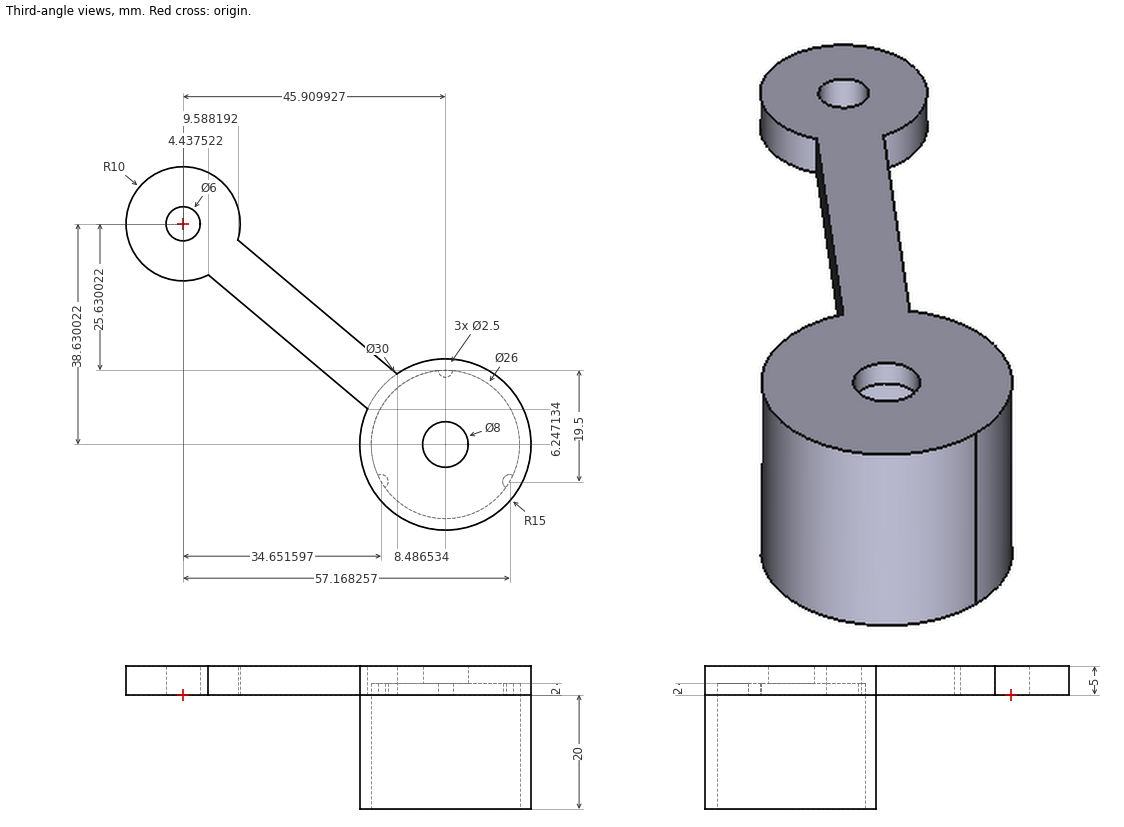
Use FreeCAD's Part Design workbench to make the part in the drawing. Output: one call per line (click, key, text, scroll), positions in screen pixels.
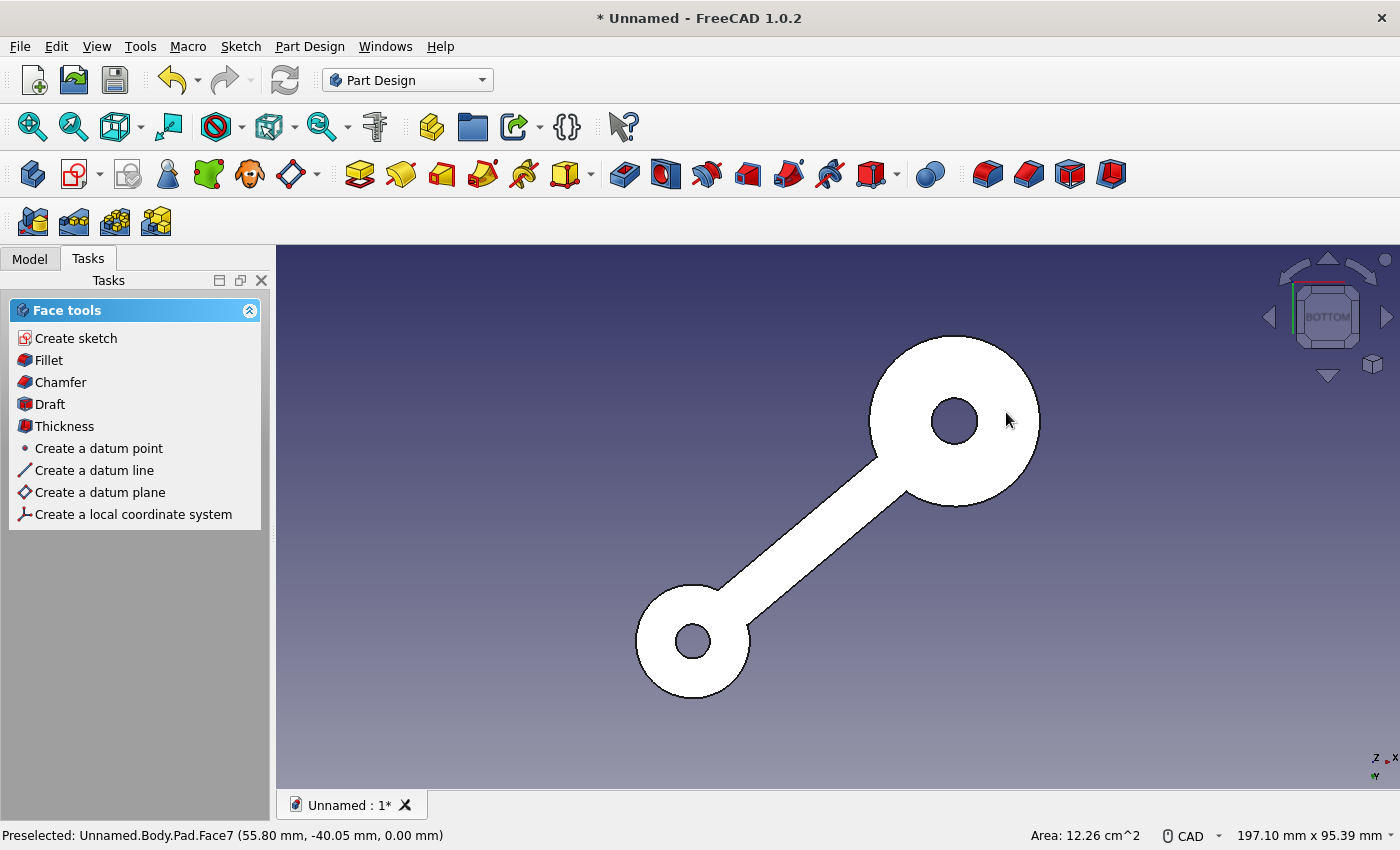
click(74, 174)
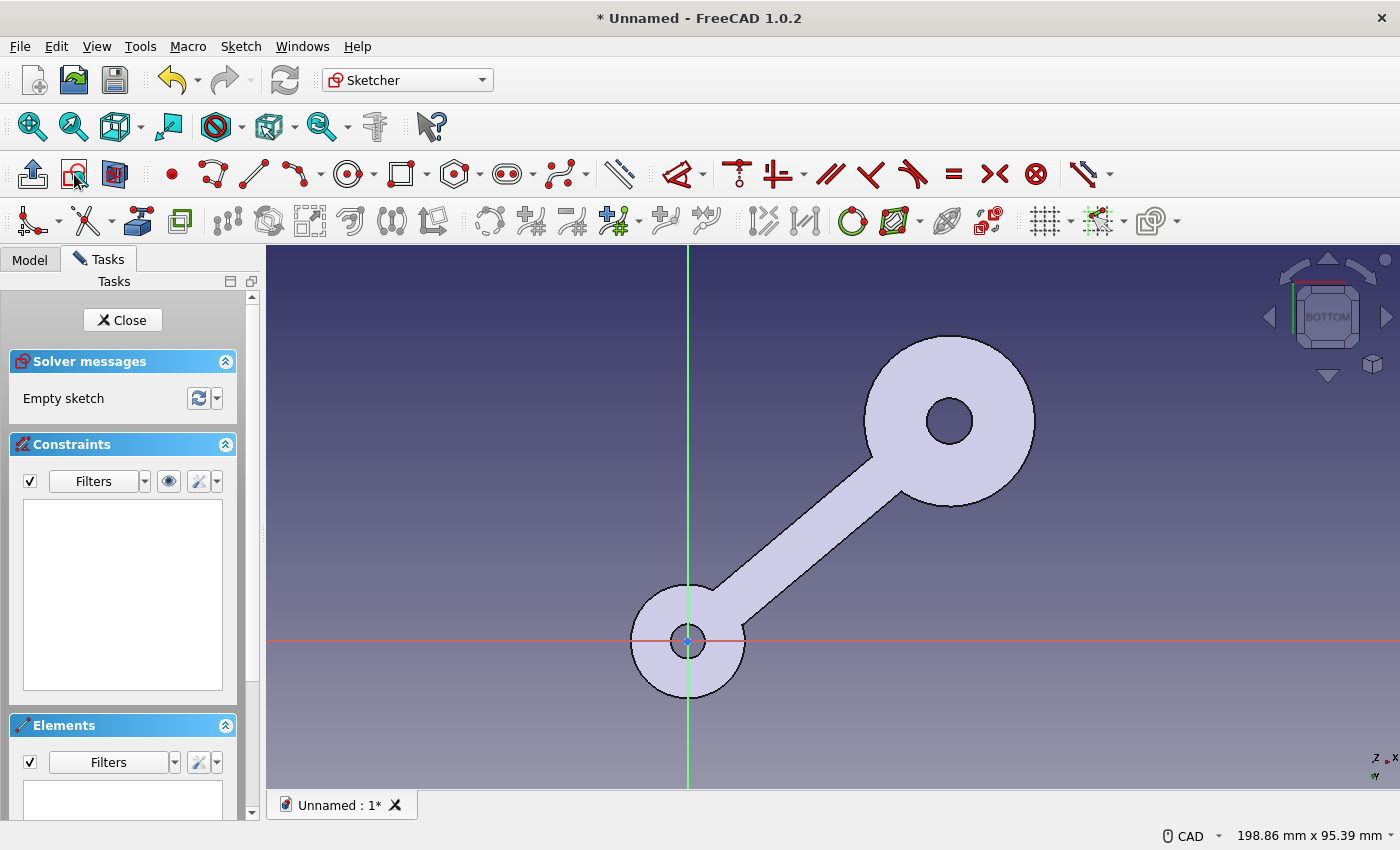
click(348, 174)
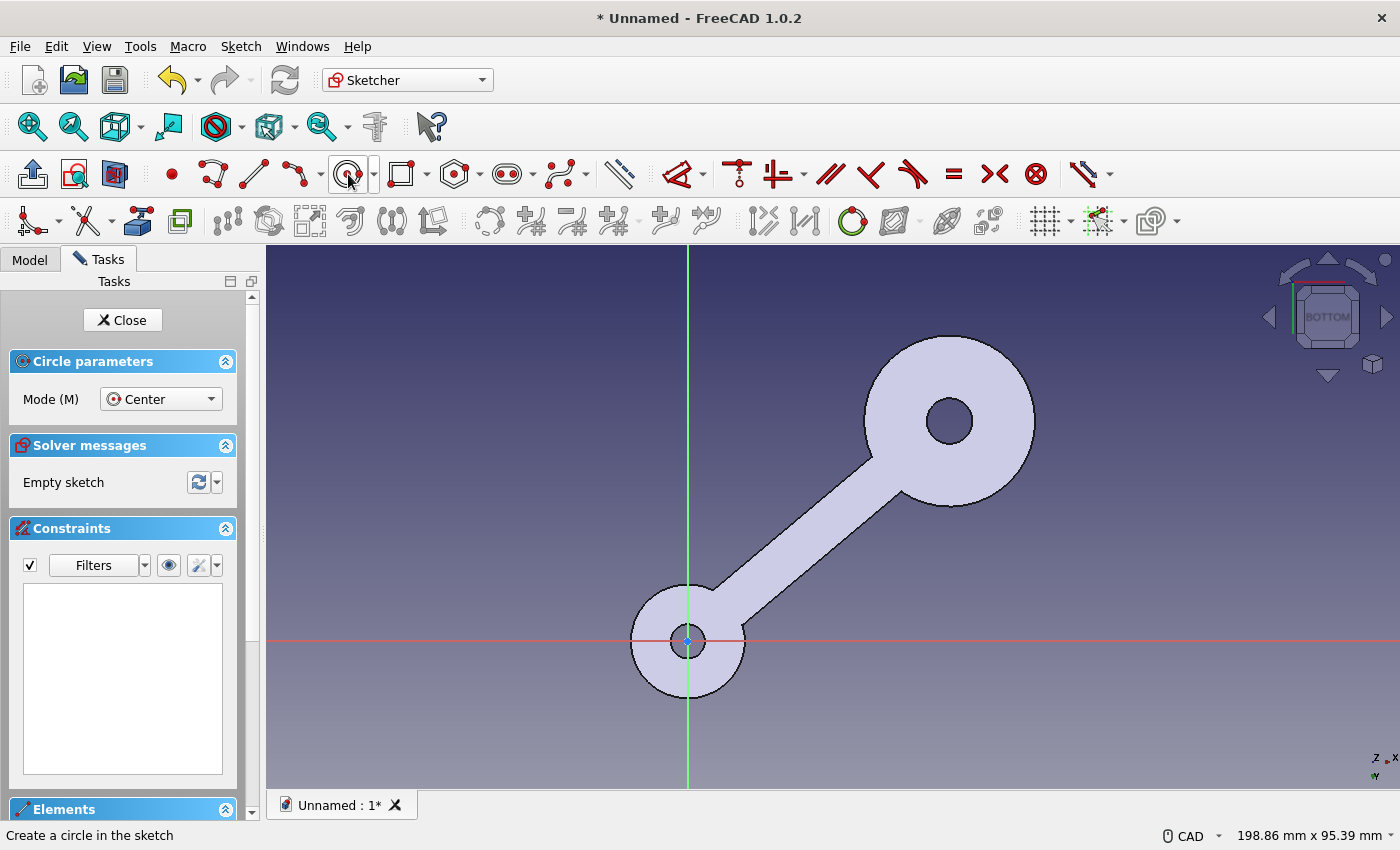
click(950, 421)
move(1002, 369)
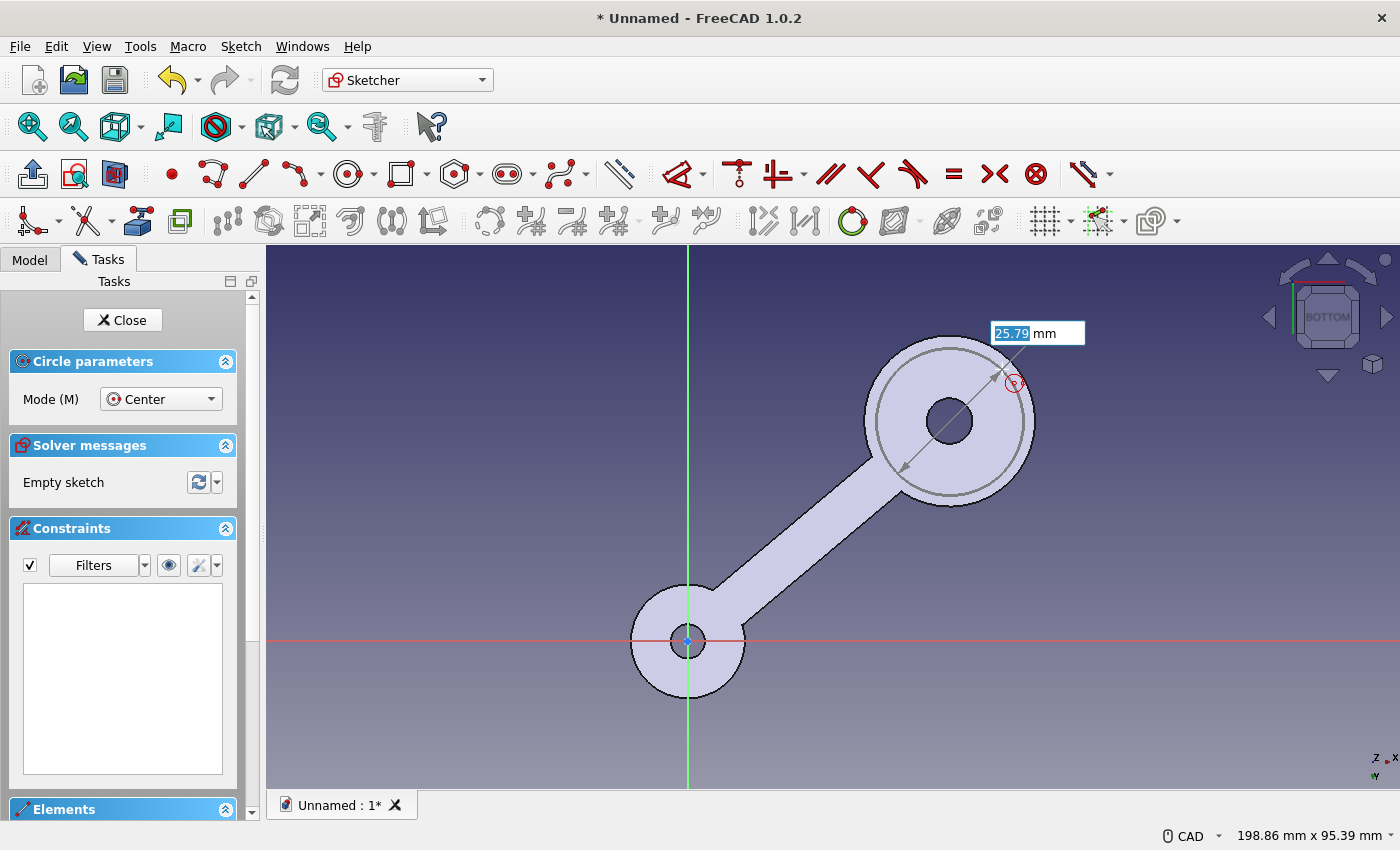
text(26)
key(Return)
key(Escape)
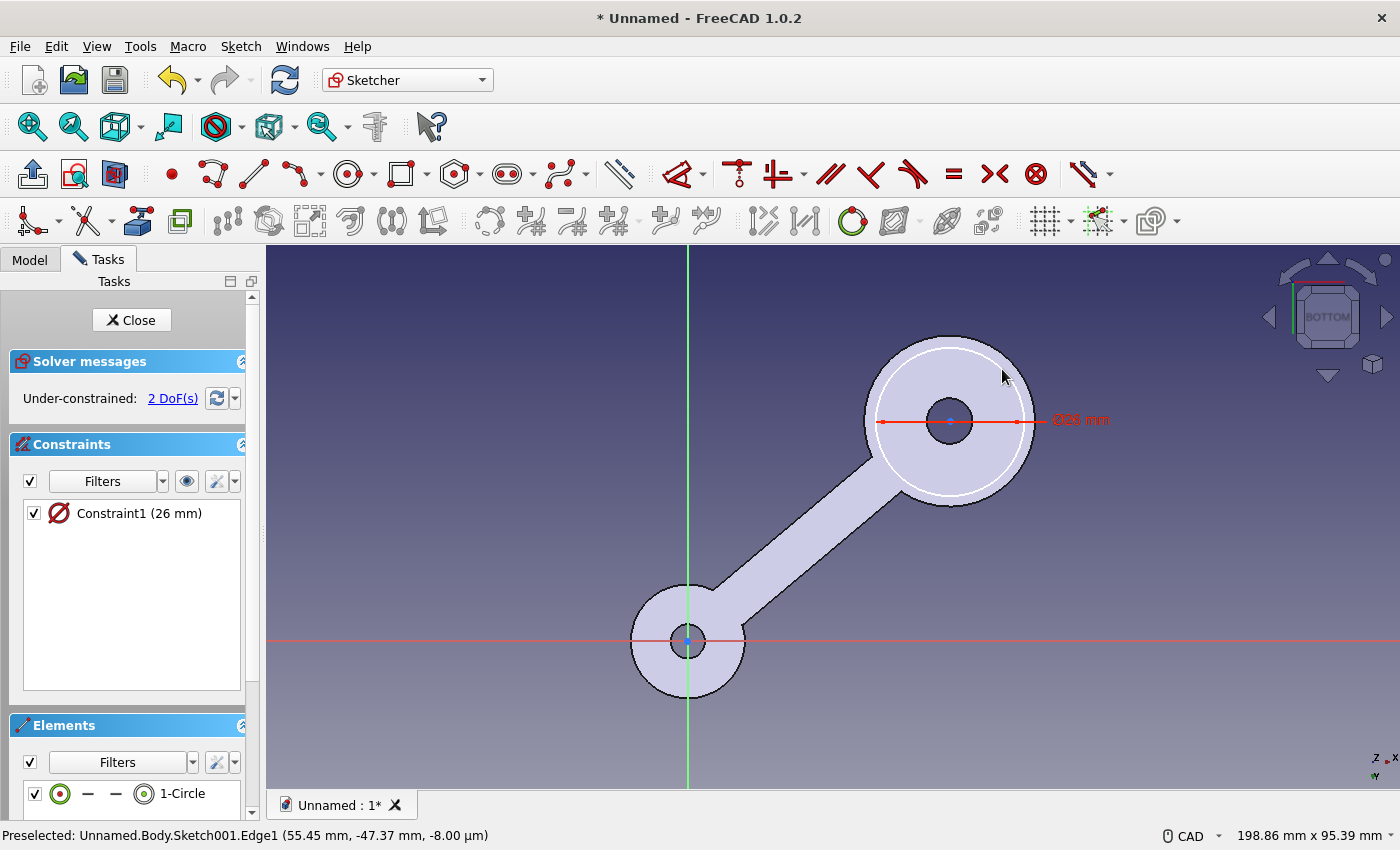
key(d)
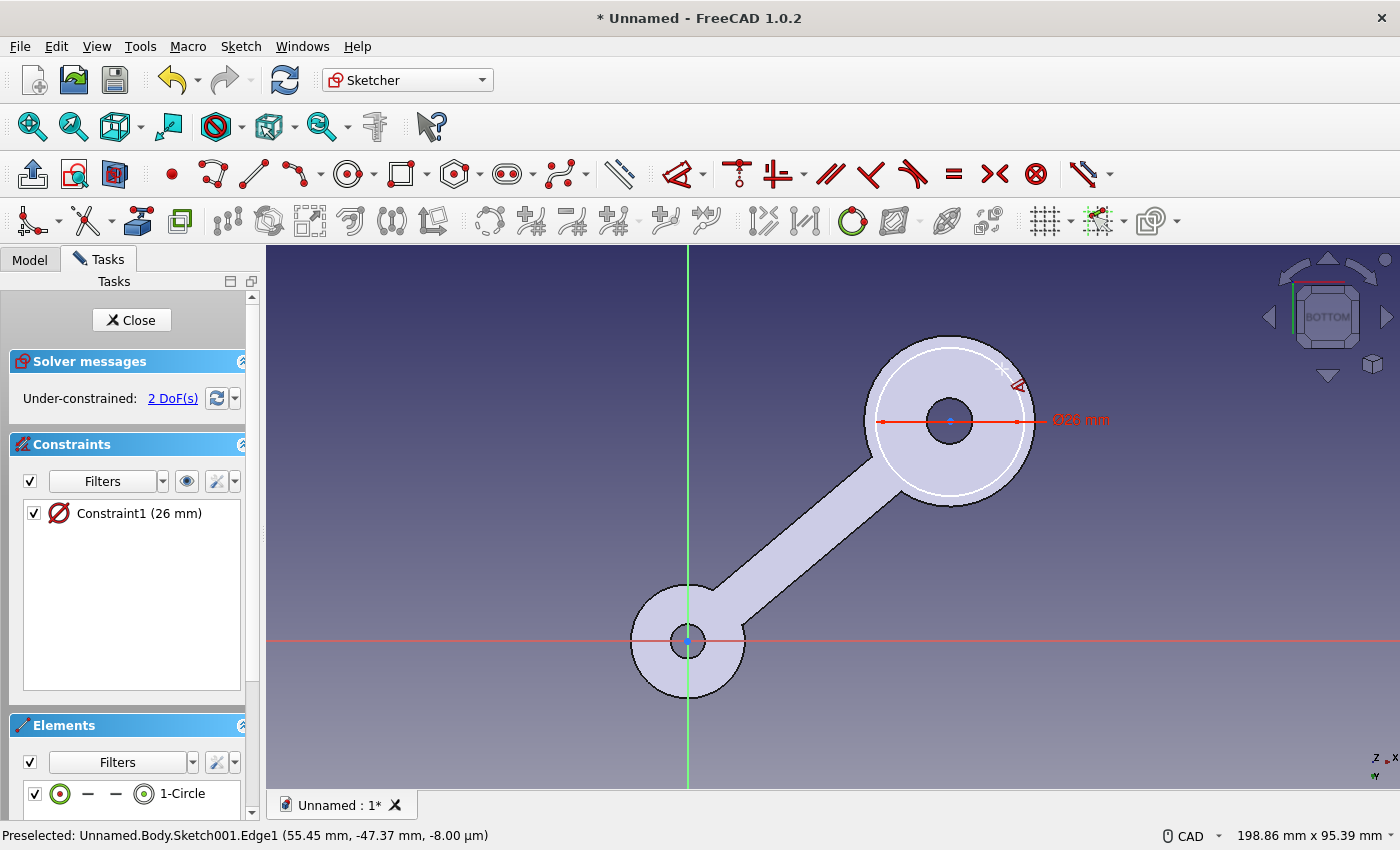
click(950, 422)
click(819, 675)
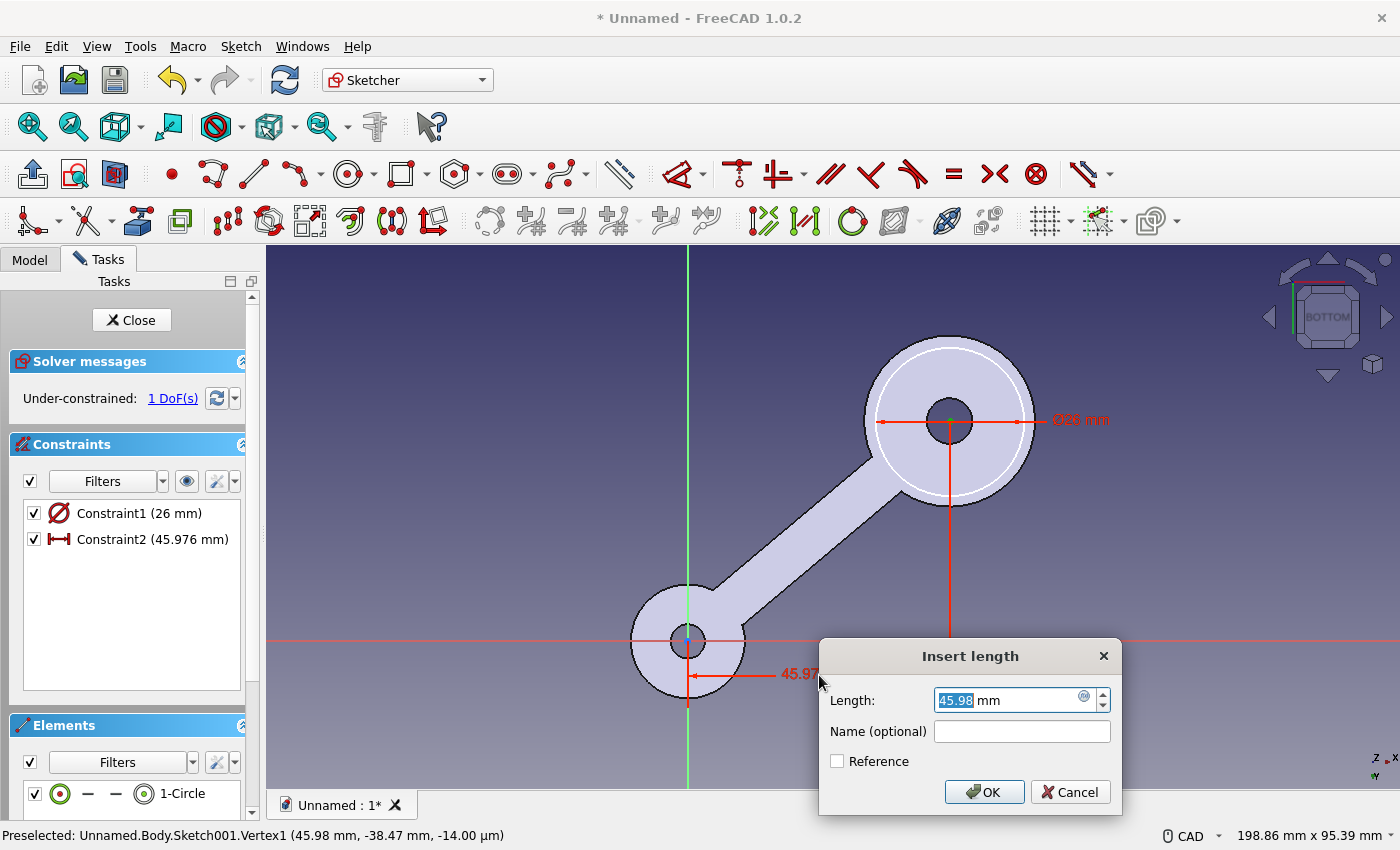
text(45.909927)
key(Return)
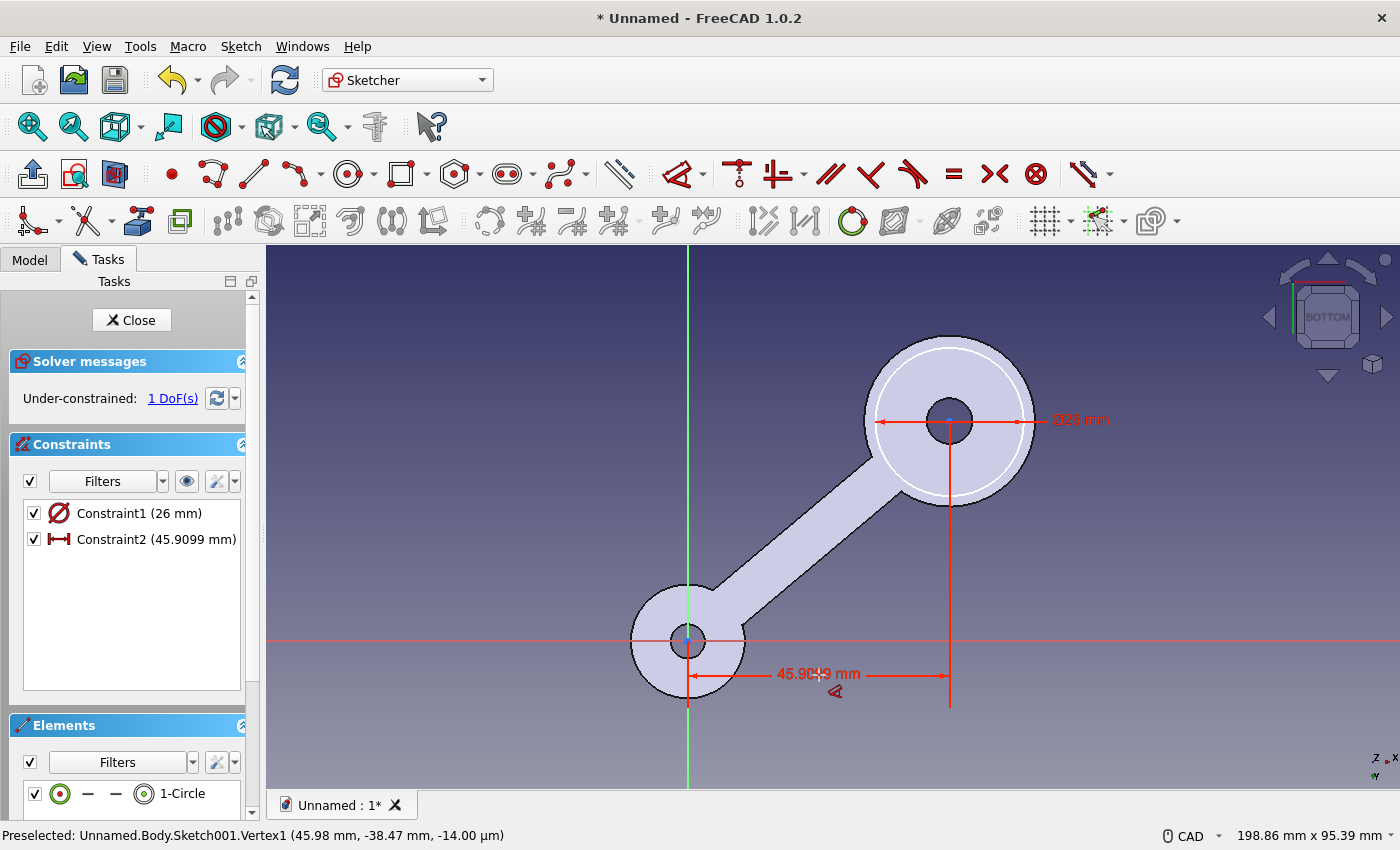
click(950, 422)
click(654, 532)